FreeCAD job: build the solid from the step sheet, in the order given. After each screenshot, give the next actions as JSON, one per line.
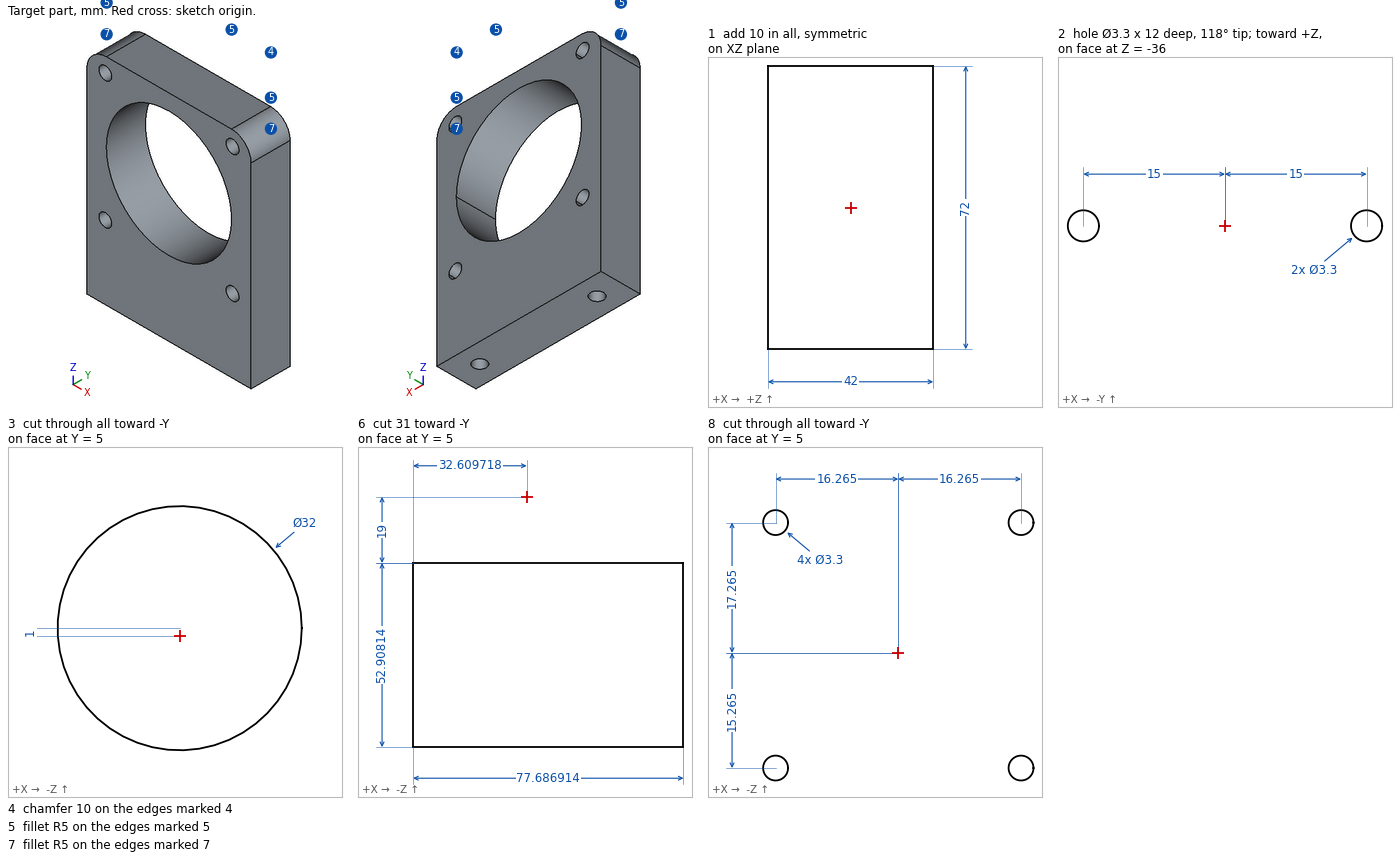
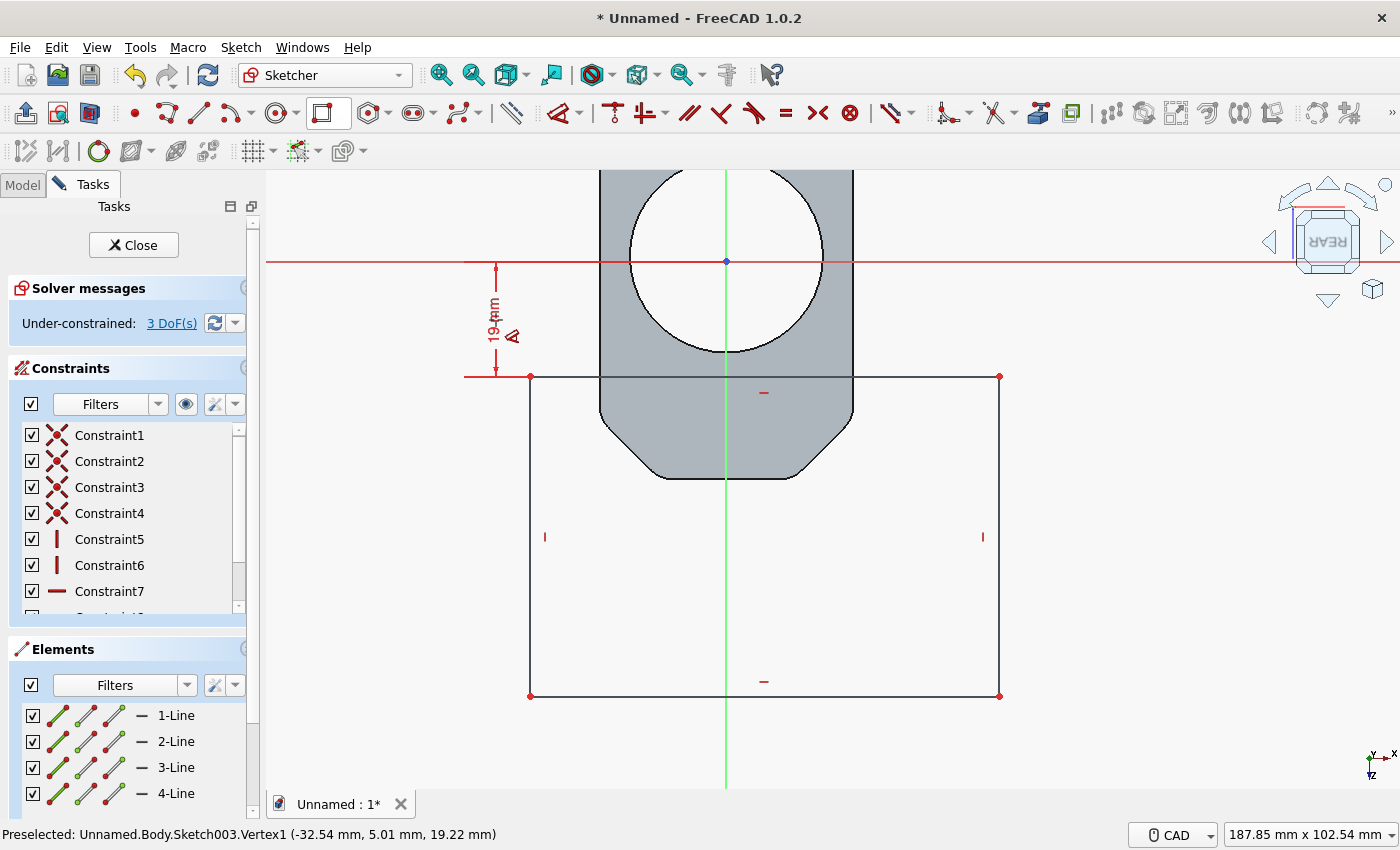
{"action": "left_click", "coordinate": [530, 473]}
{"action": "left_click", "coordinate": [496, 537]}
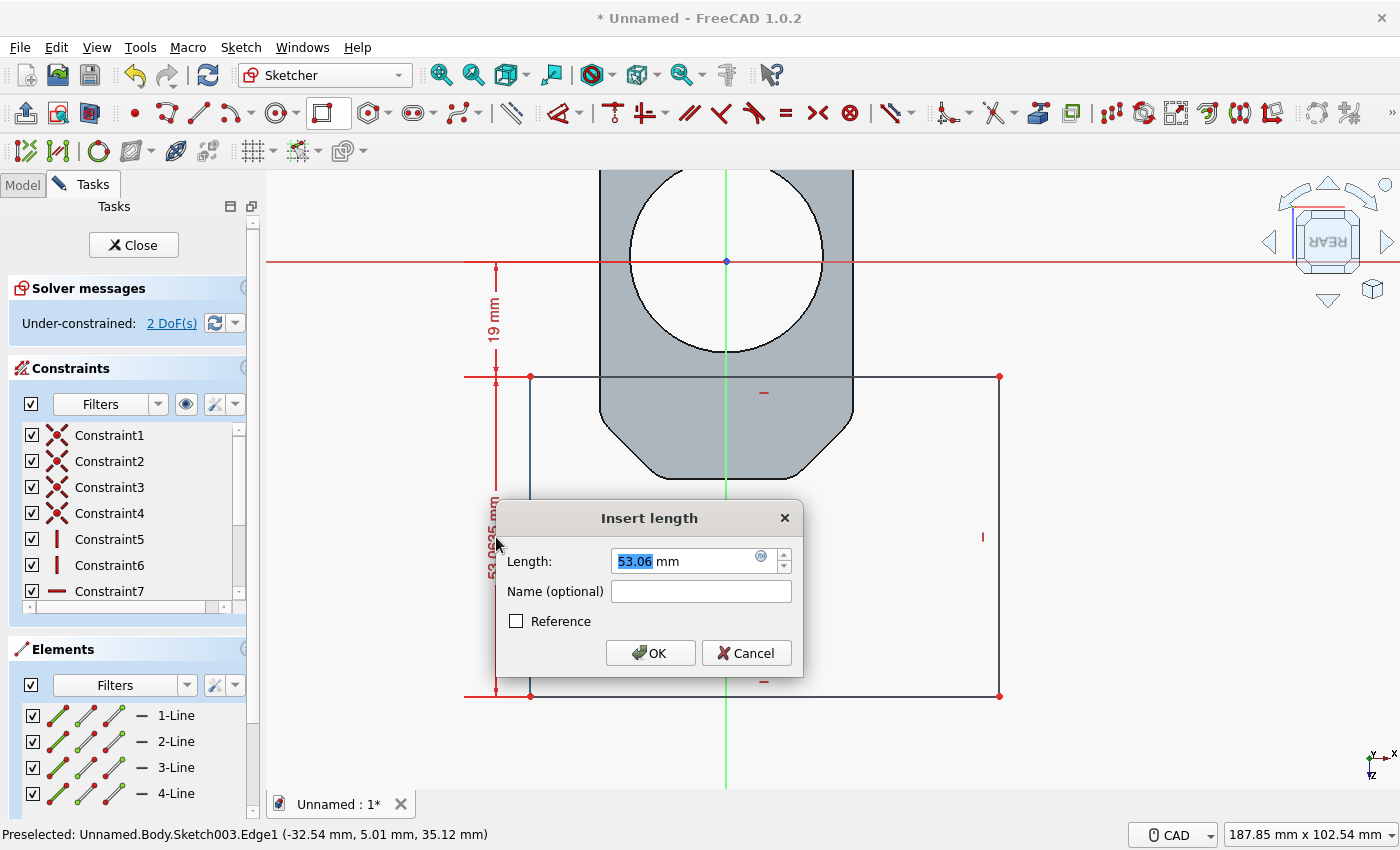
{"action": "type", "text": "52.90814"}
{"action": "key", "text": "Return"}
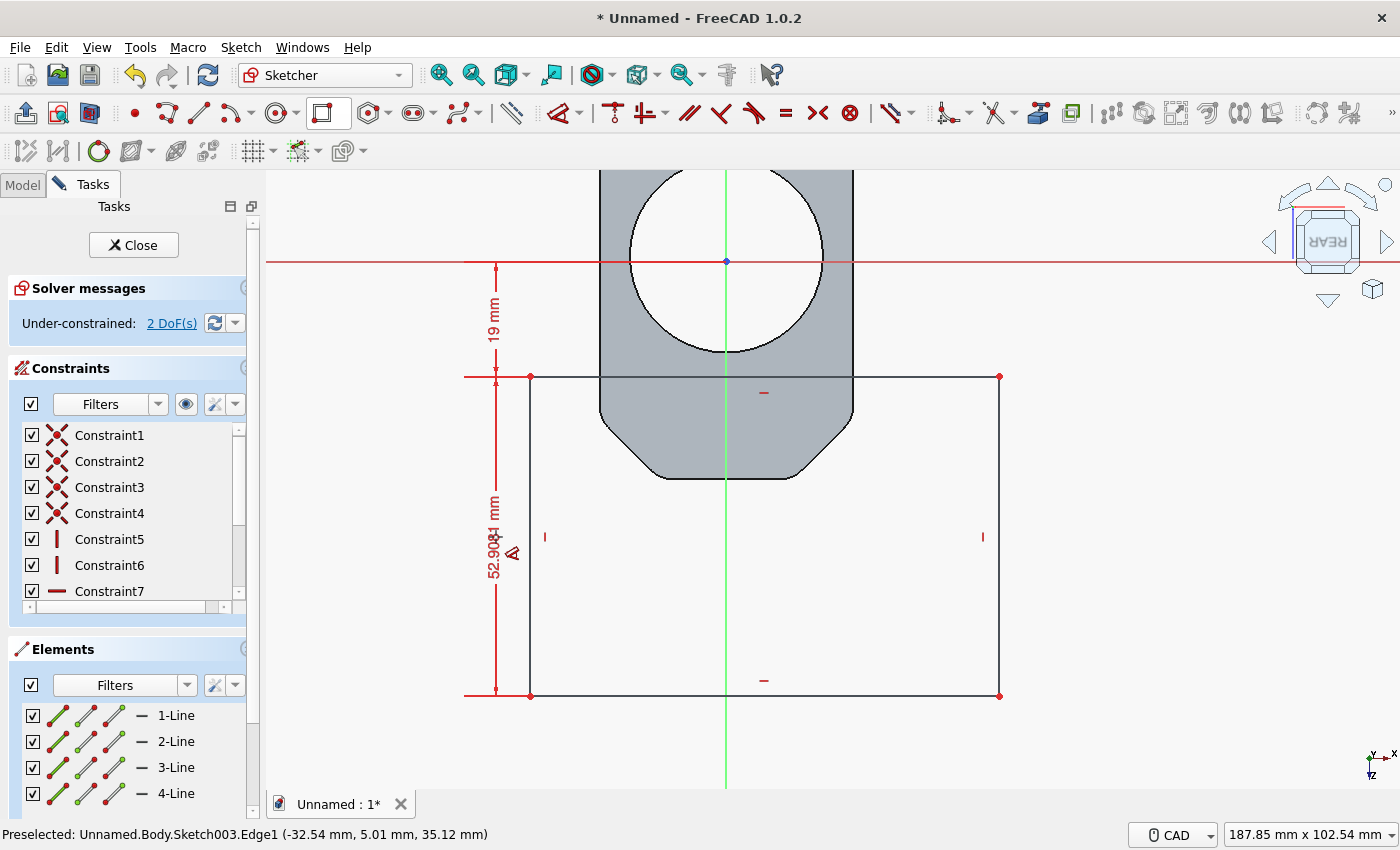
{"action": "left_click", "coordinate": [671, 696]}
{"action": "left_click", "coordinate": [765, 730]}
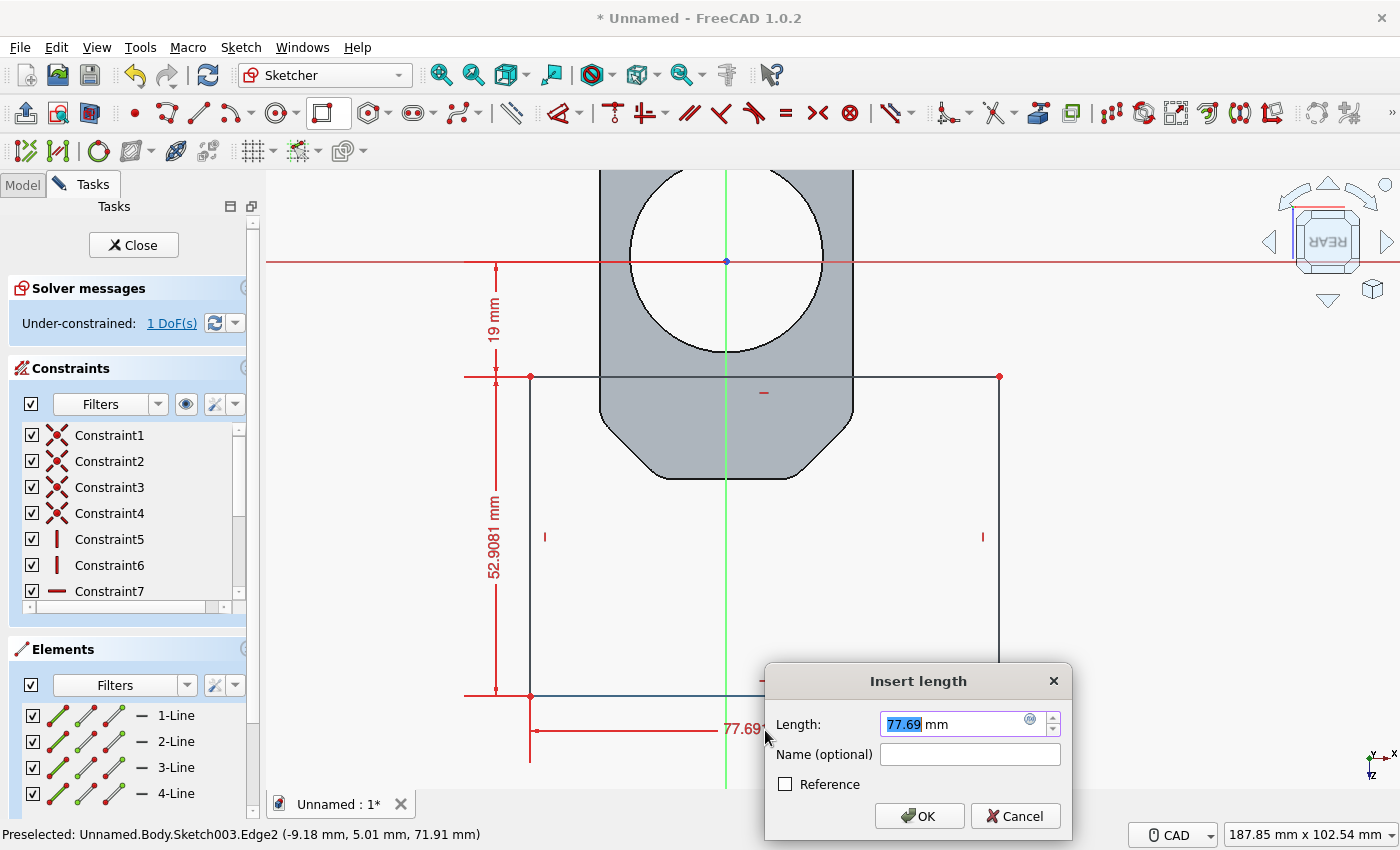
{"action": "type", "text": "77.686914"}
{"action": "key", "text": "Return"}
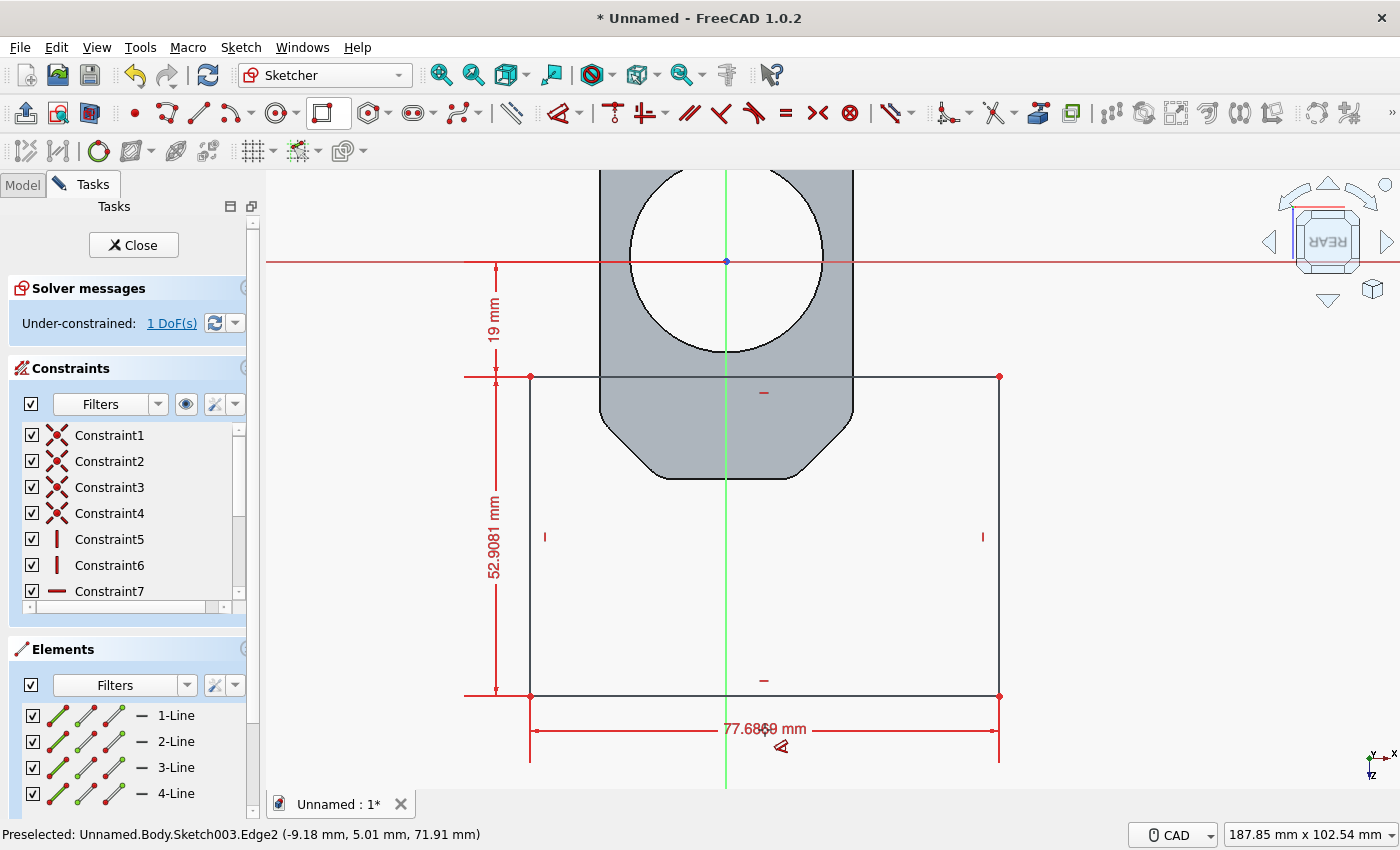
{"action": "left_click", "coordinate": [530, 377]}
{"action": "left_click", "coordinate": [628, 228]}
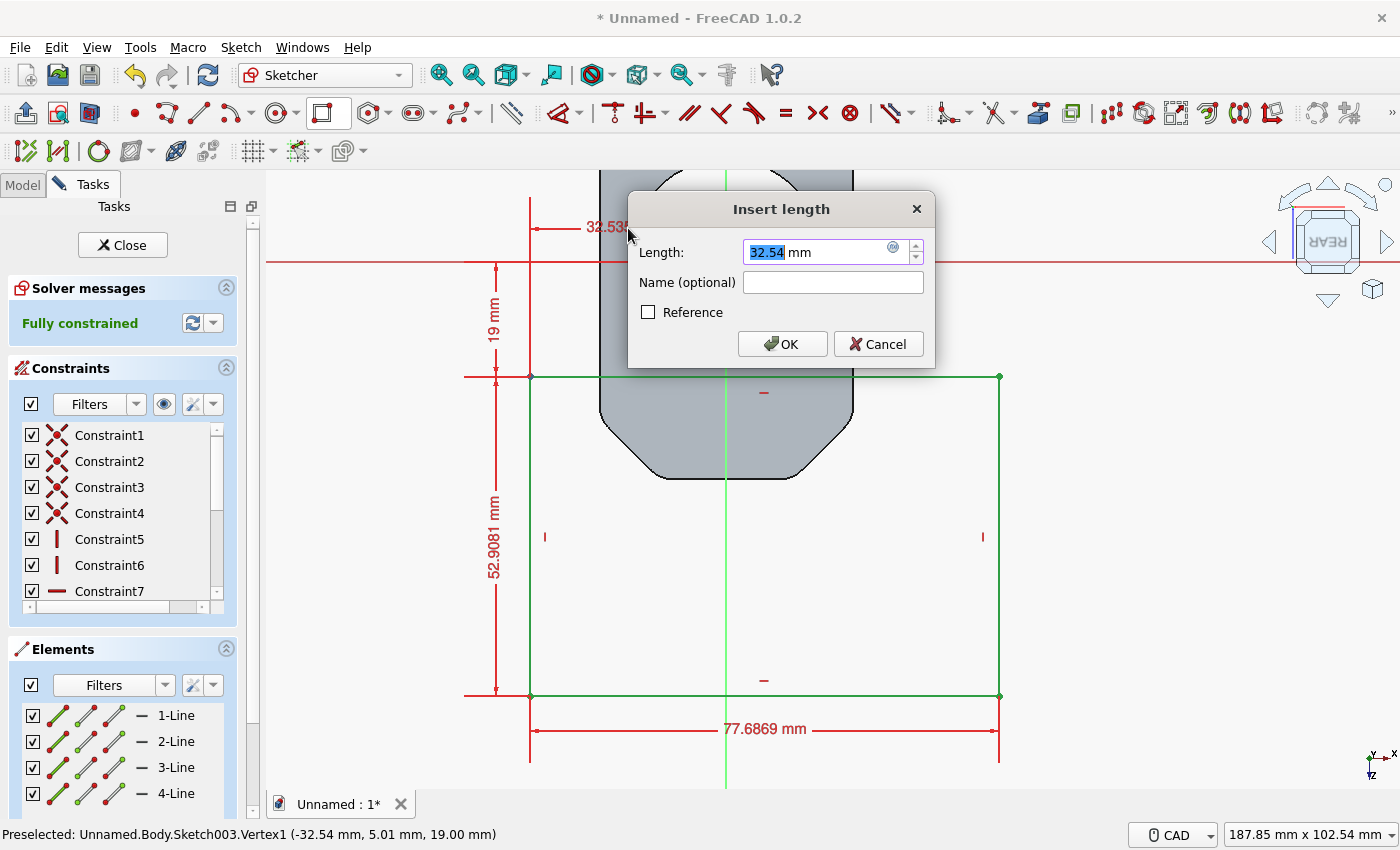
{"action": "type", "text": "32.609718"}
{"action": "key", "text": "Return"}
{"action": "key", "text": "Escape"}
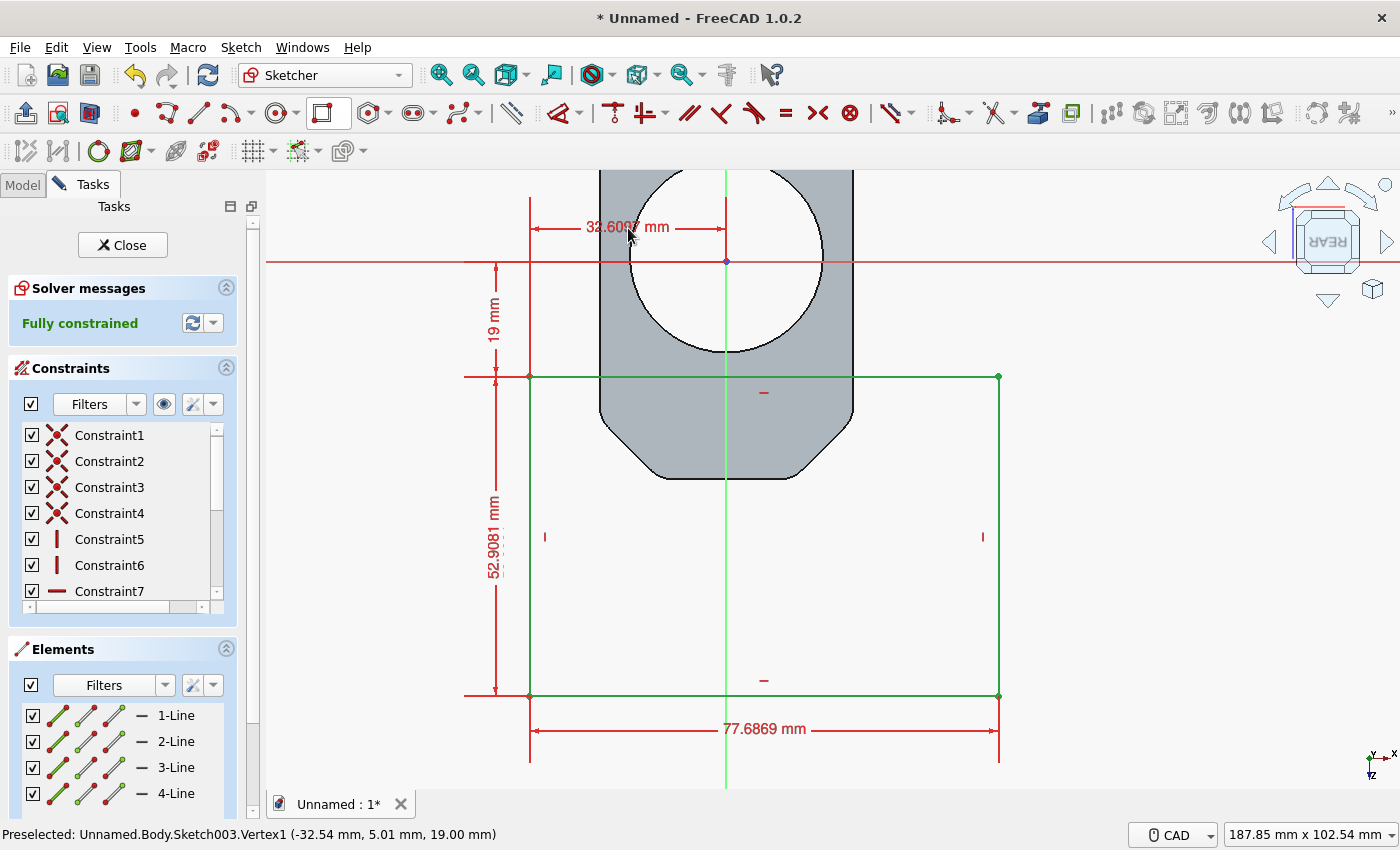
{"action": "left_click", "coordinate": [123, 245]}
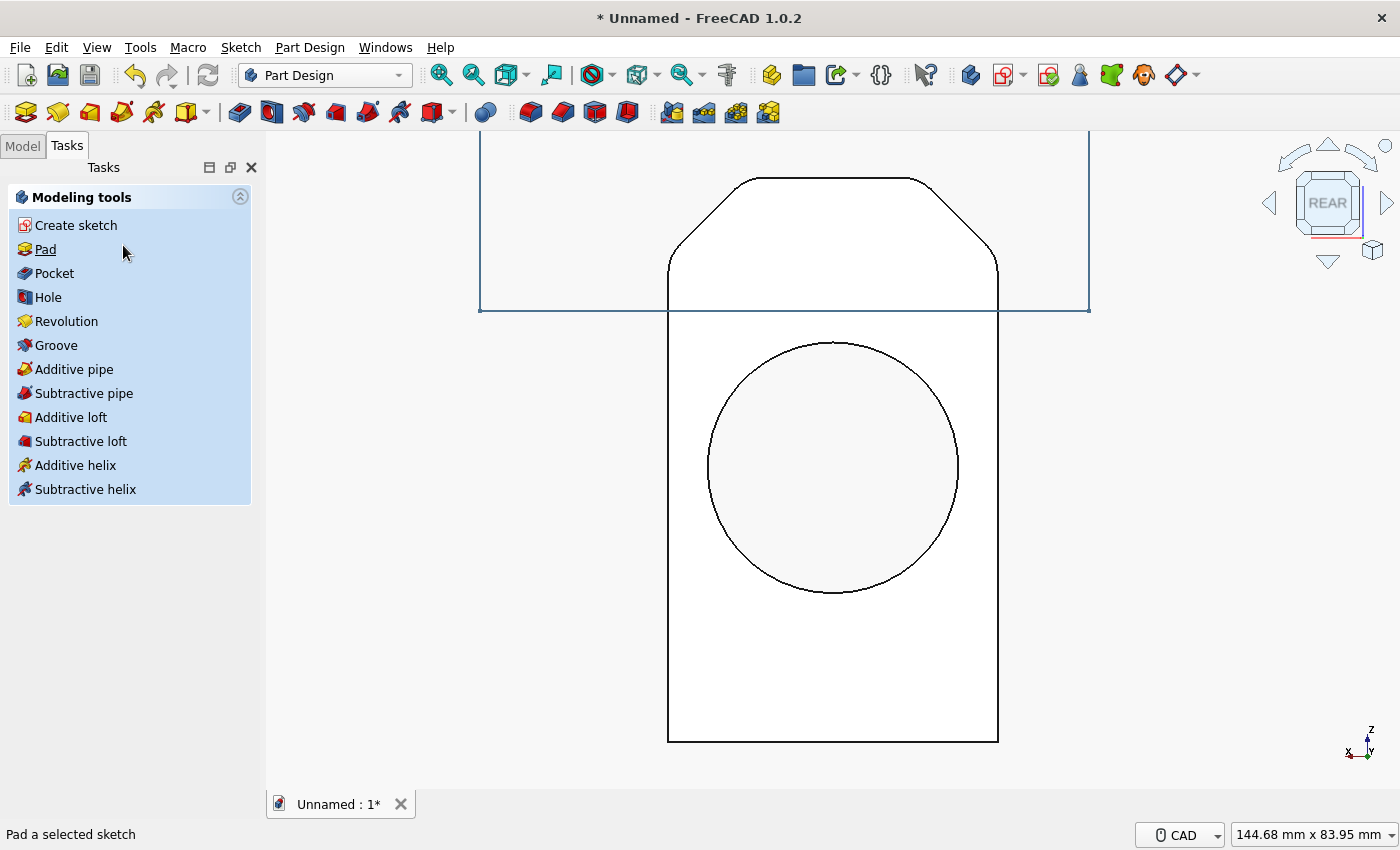
{"action": "left_click", "coordinate": [240, 112]}